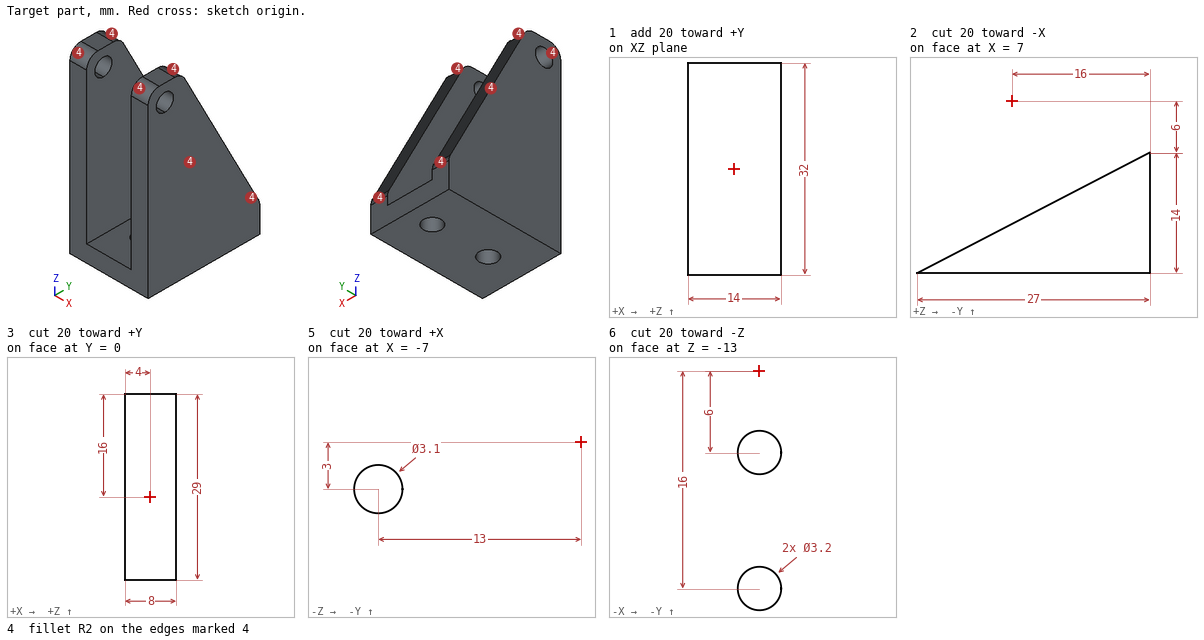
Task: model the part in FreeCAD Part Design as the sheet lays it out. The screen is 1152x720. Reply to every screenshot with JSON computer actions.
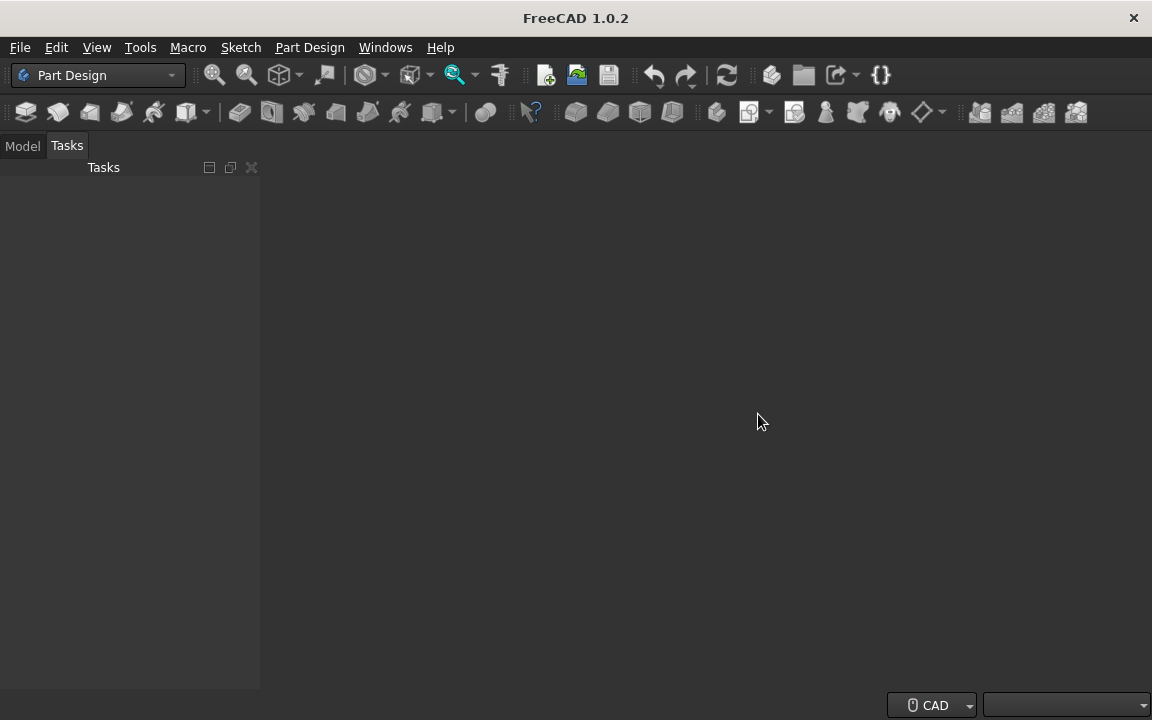
{"action": "left_click", "coordinate": [546, 76]}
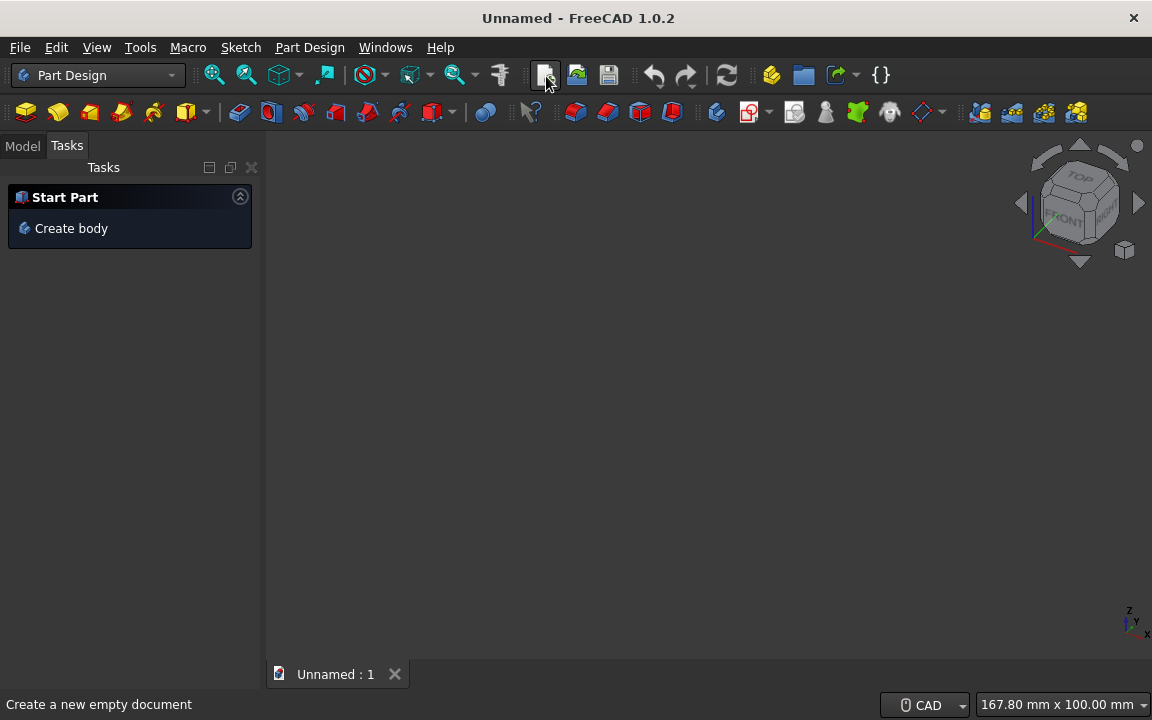
{"action": "left_click", "coordinate": [750, 112]}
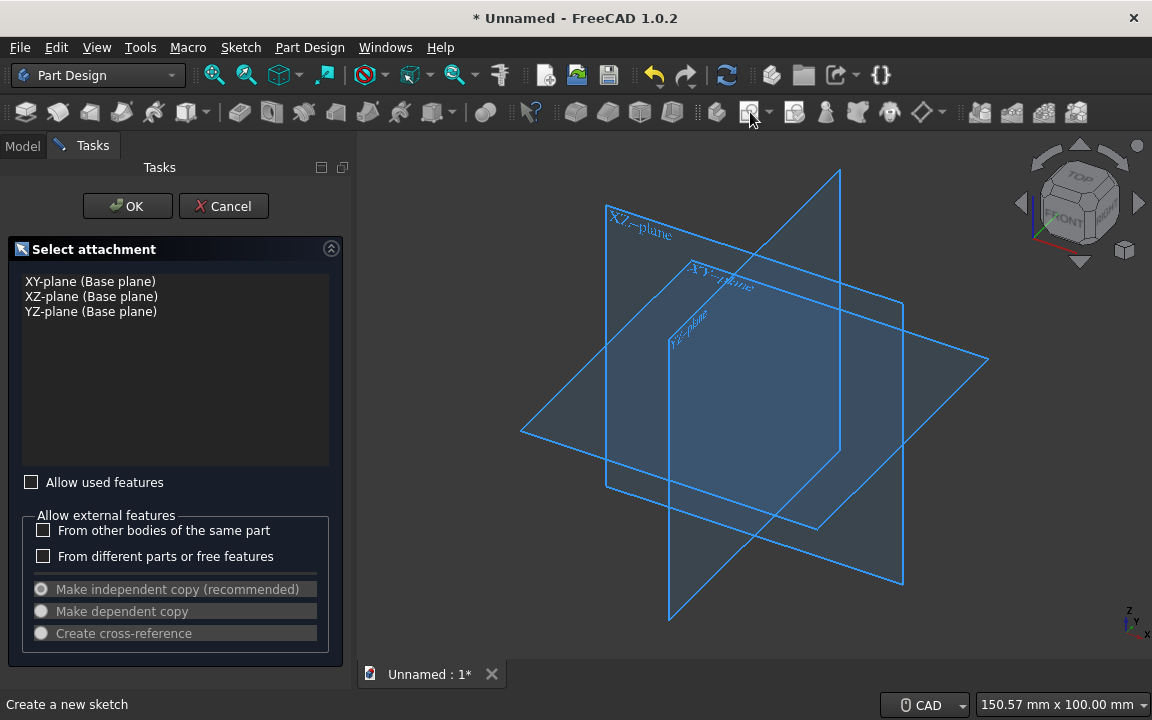
{"action": "left_click", "coordinate": [82, 296]}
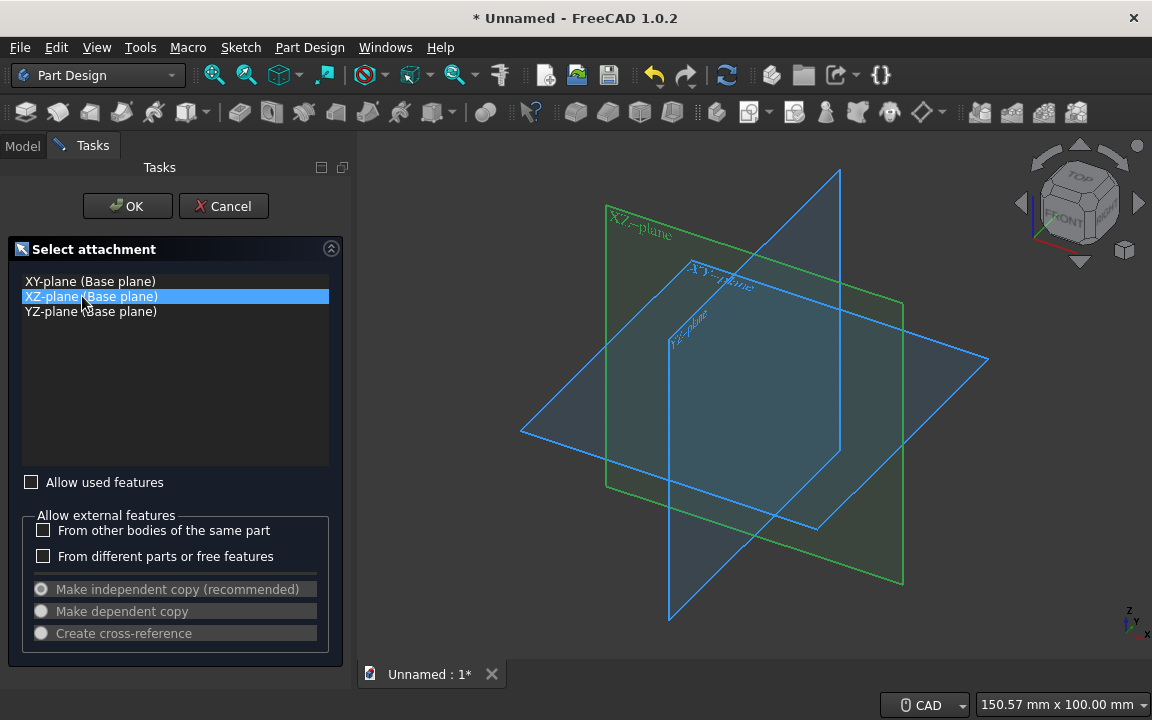
{"action": "left_click", "coordinate": [128, 206]}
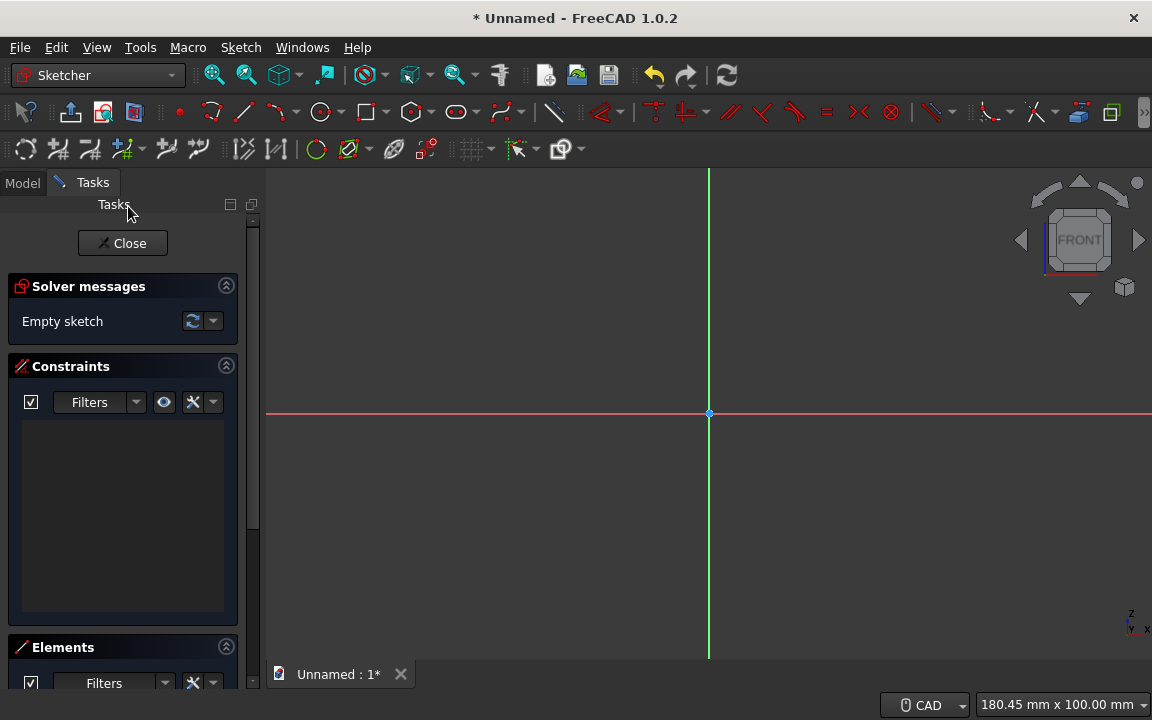
{"action": "scroll", "coordinate": [792, 414], "scroll_direction": "up", "scroll_amount": 3}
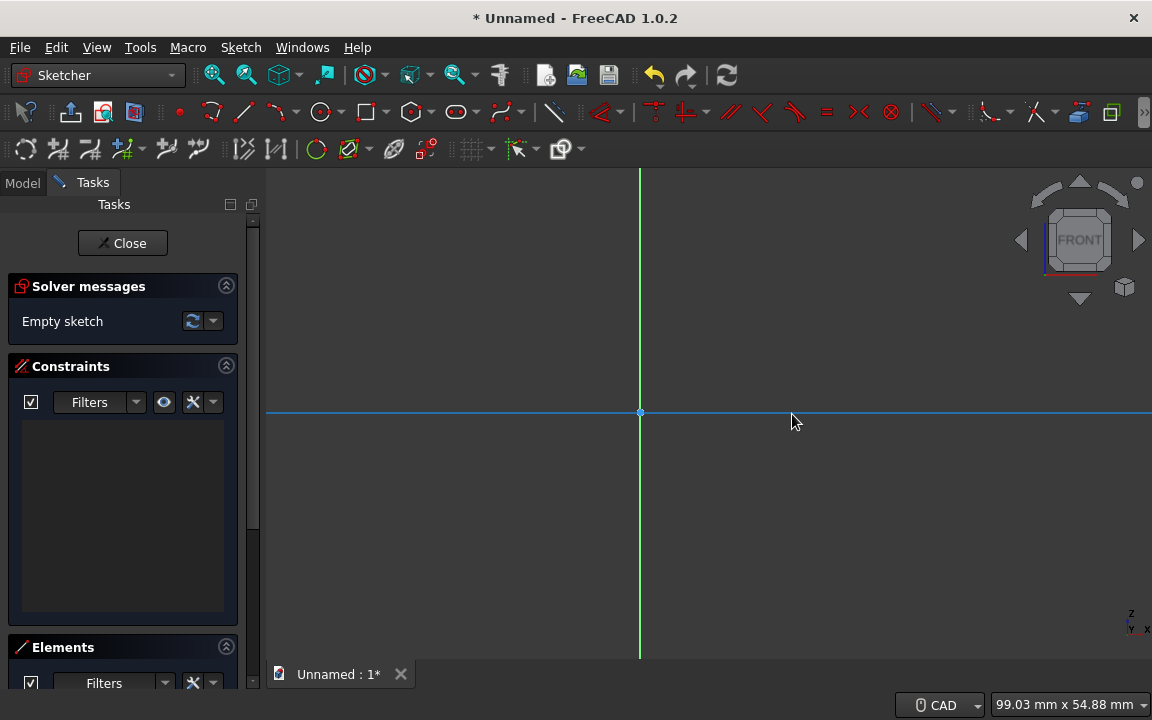
{"action": "key", "text": "g v"}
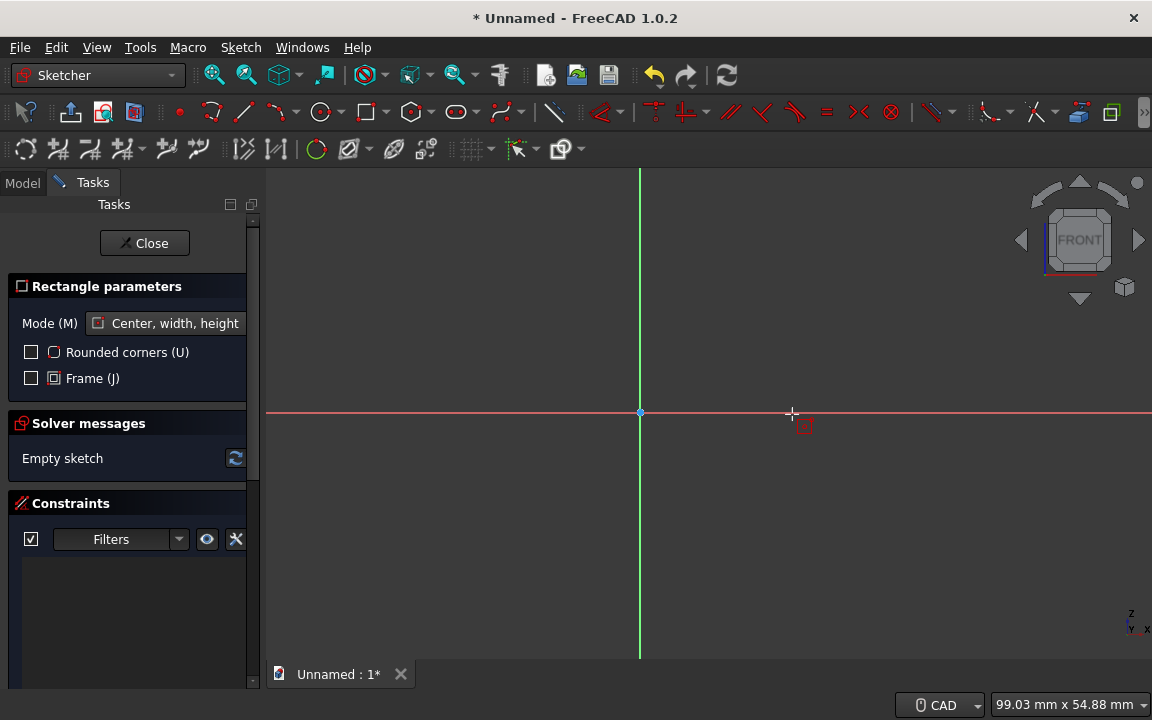
{"action": "left_click", "coordinate": [640, 413]}
{"action": "mouse_move", "coordinate": [703, 270]}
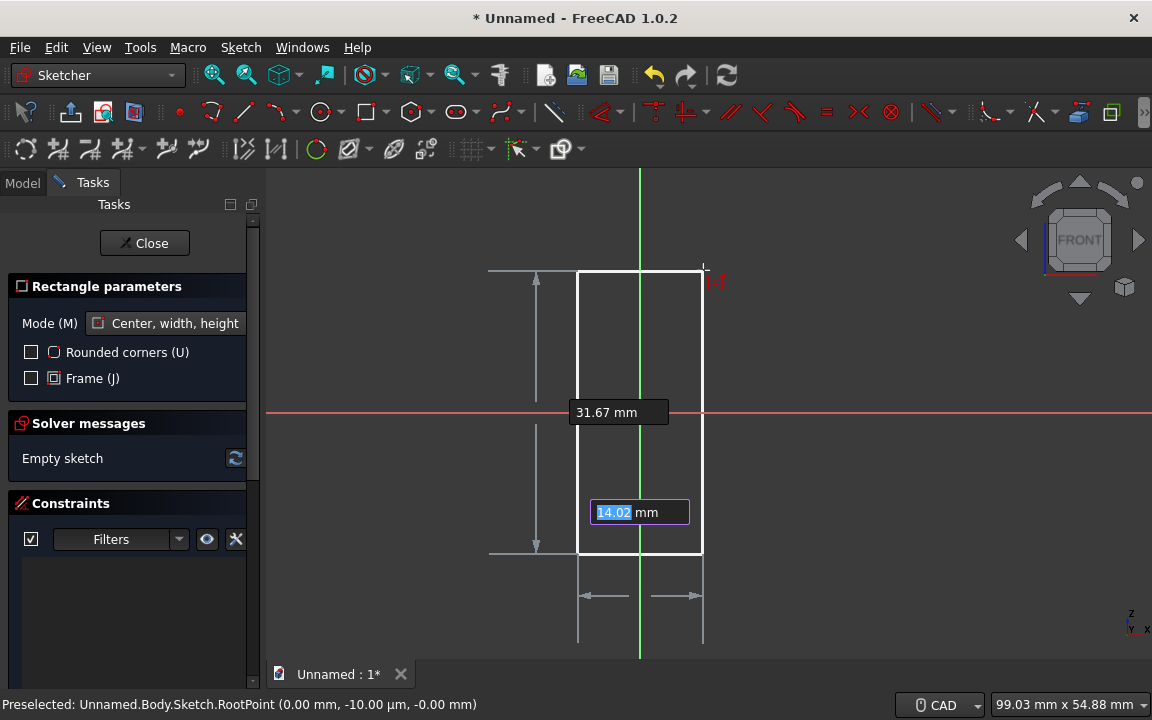
{"action": "type", "text": "14"}
{"action": "key", "text": "Tab"}
{"action": "type", "text": "32"}
{"action": "key", "text": "Return"}
{"action": "key", "text": "Escape"}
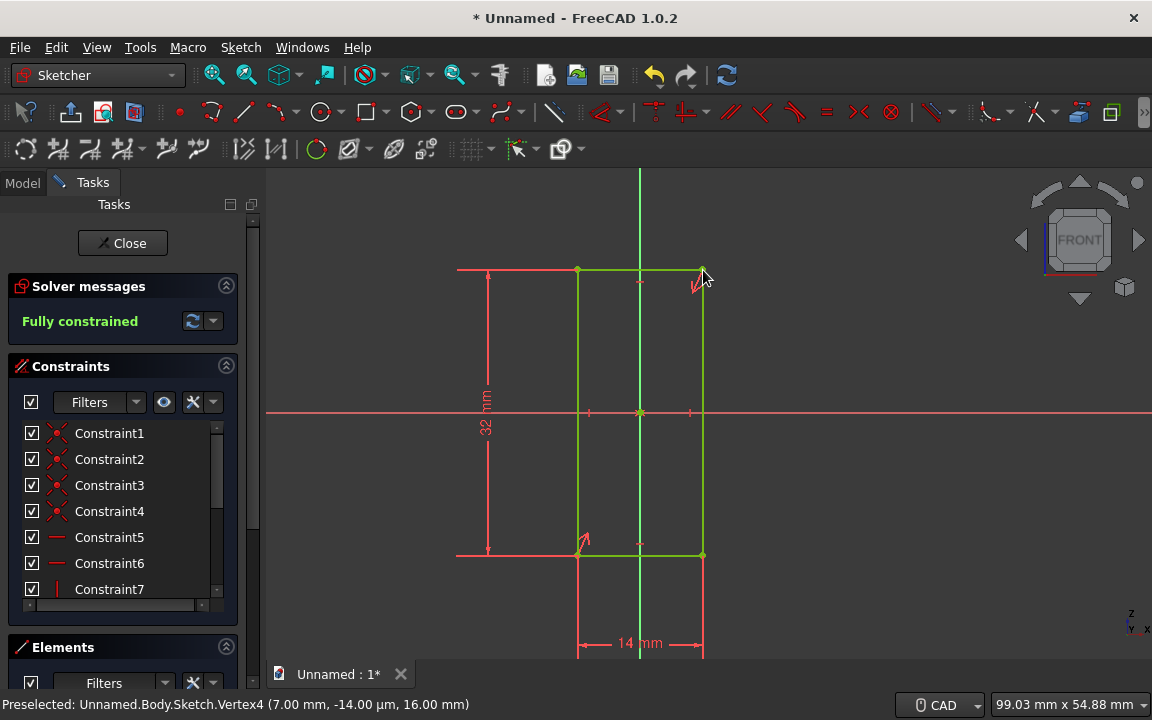
{"action": "left_click", "coordinate": [123, 243]}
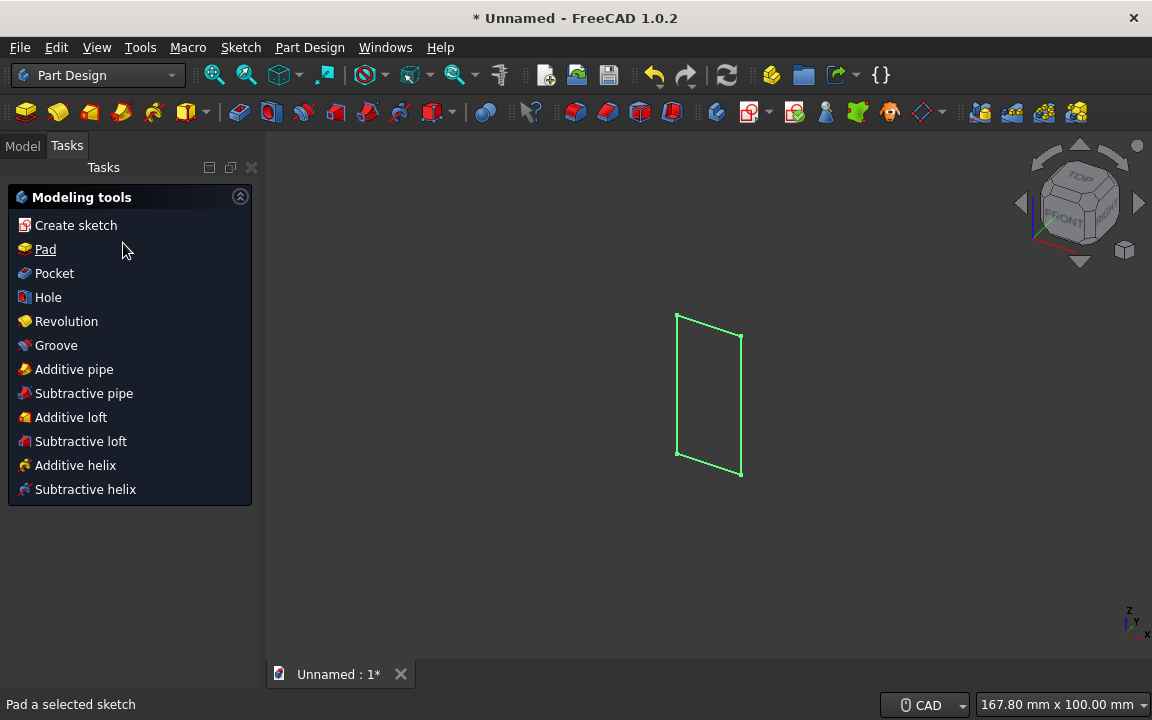
{"action": "left_click", "coordinate": [26, 112]}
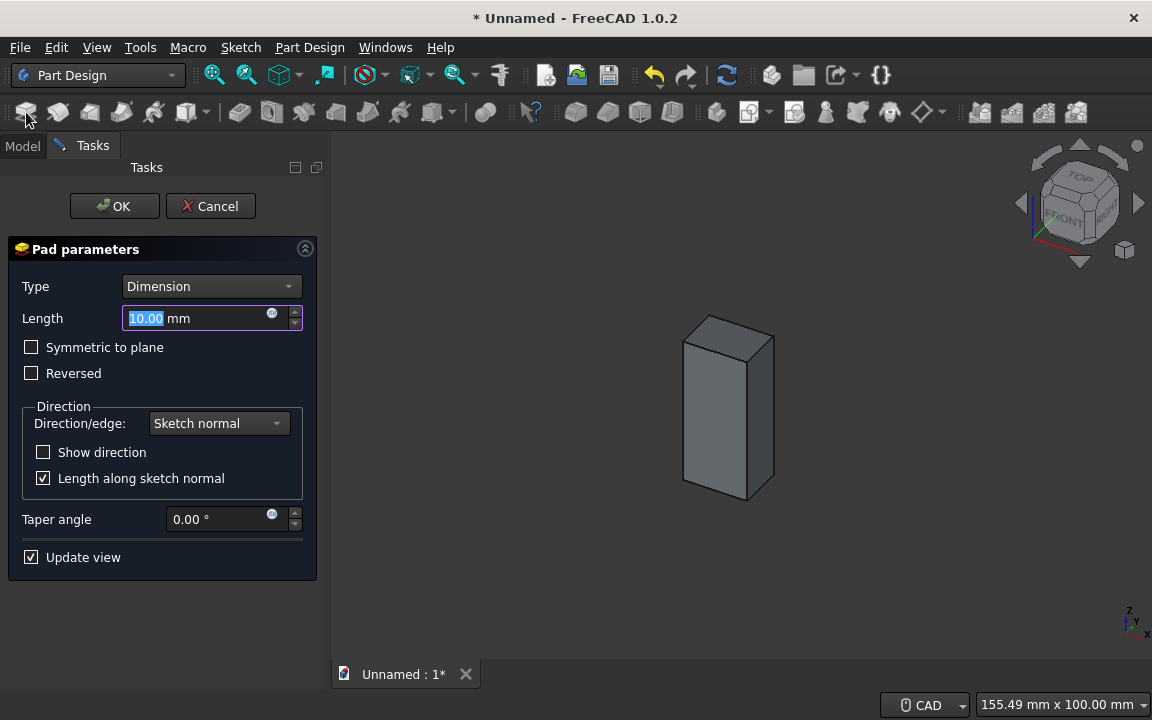
{"action": "type", "text": "20"}
{"action": "key", "text": "Tab"}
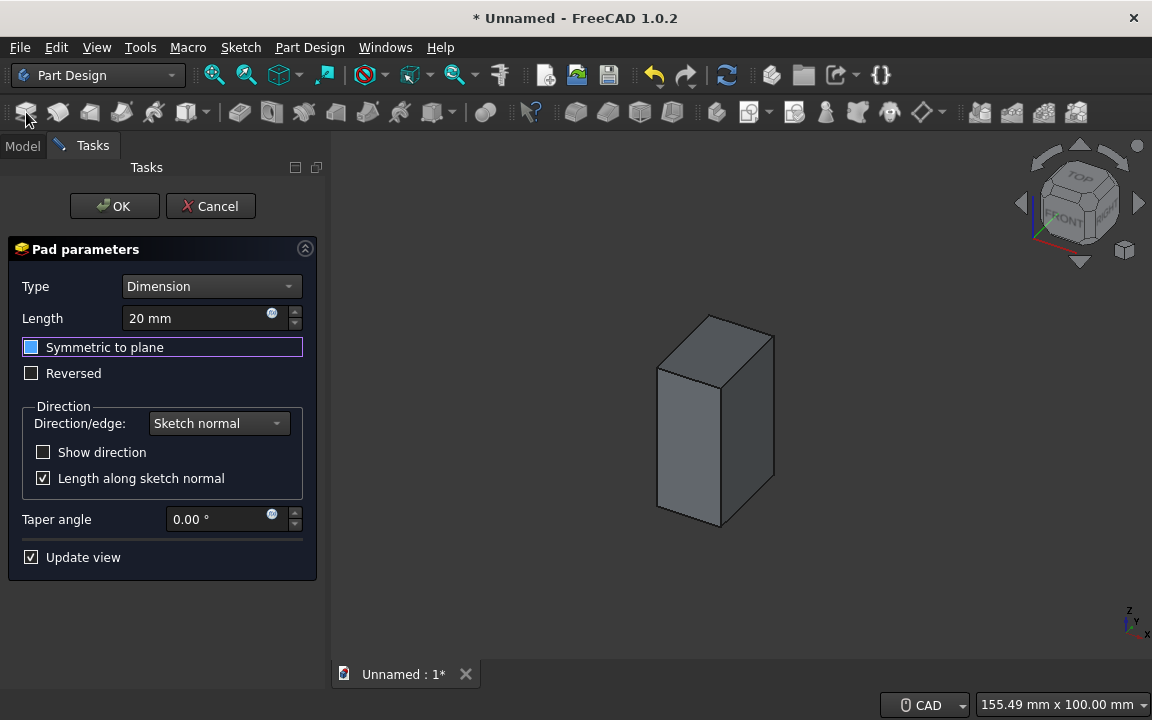
{"action": "left_click", "coordinate": [30, 373]}